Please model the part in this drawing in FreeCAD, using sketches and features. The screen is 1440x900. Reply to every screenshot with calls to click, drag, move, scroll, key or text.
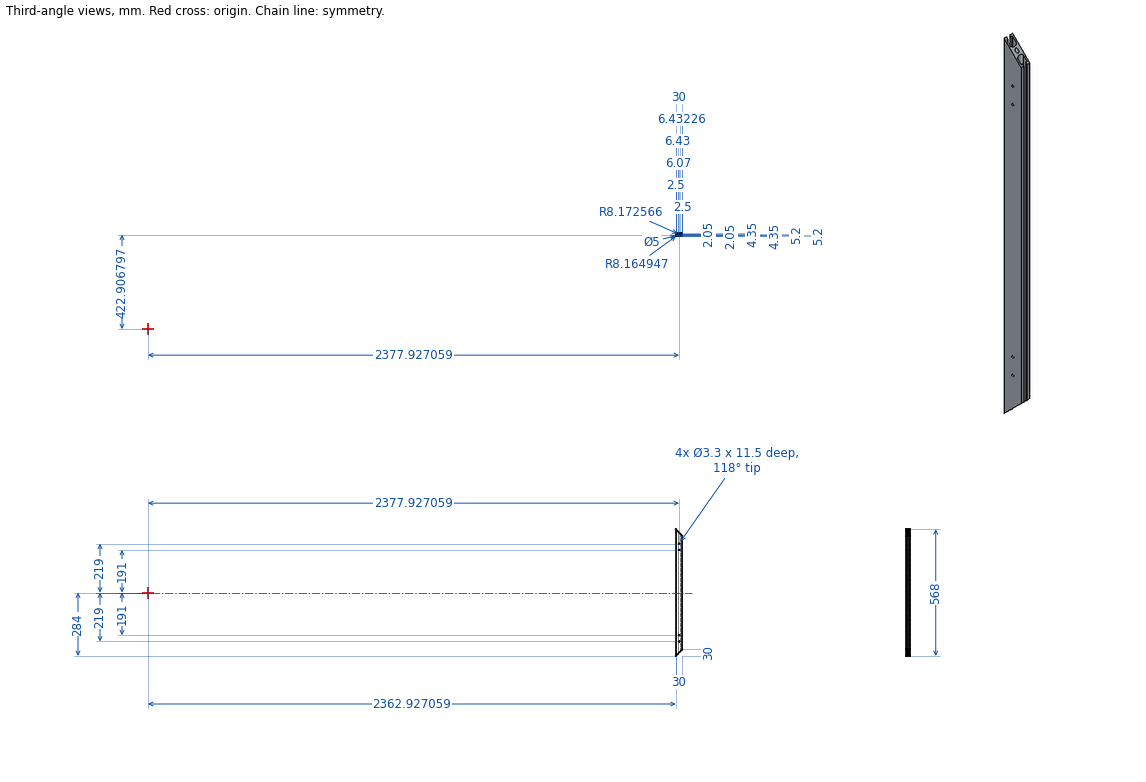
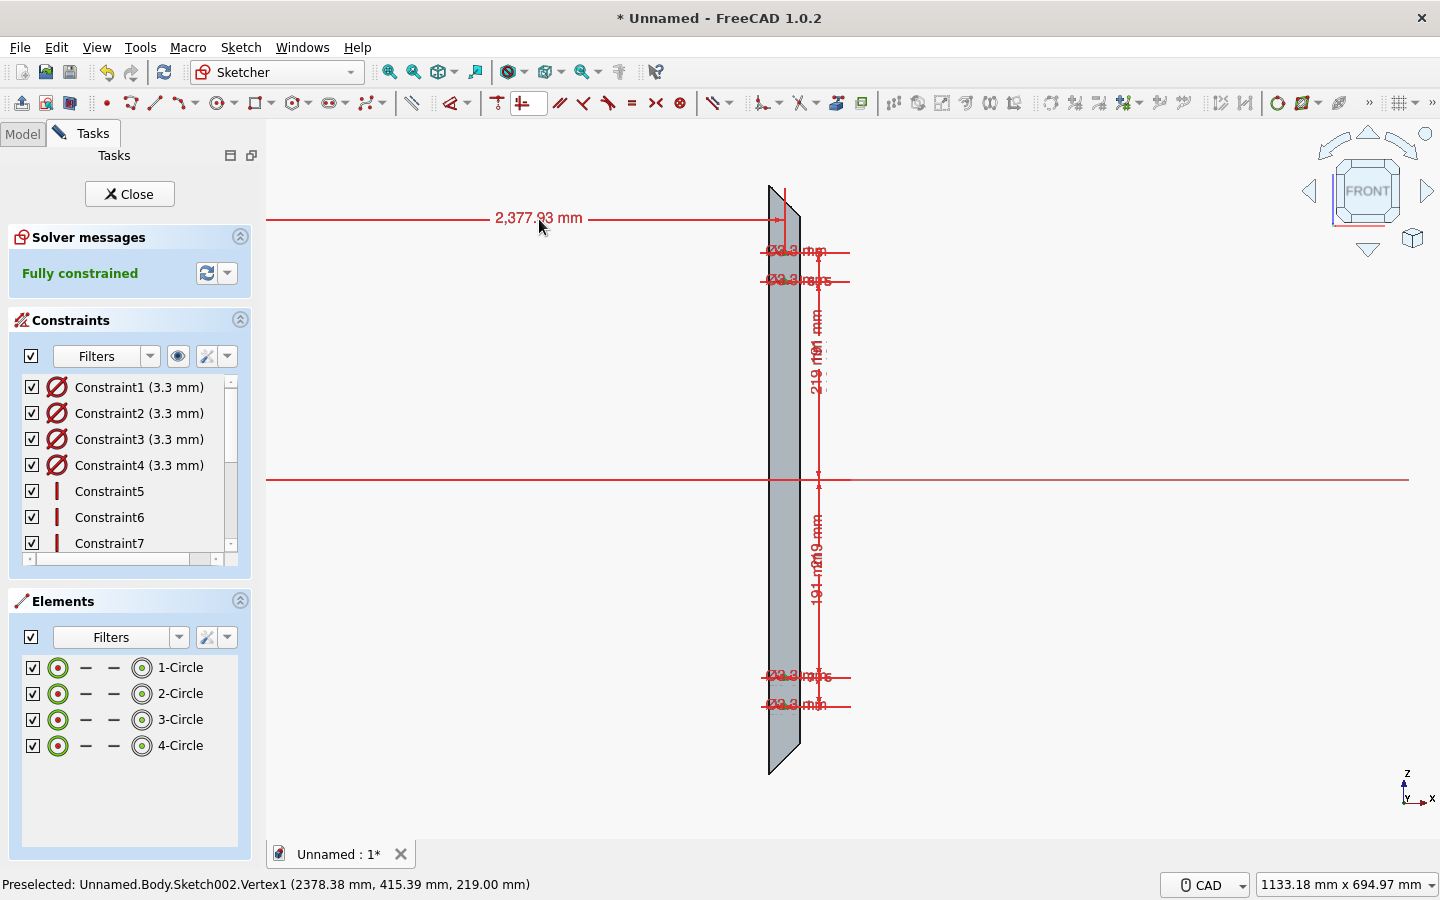
click(130, 194)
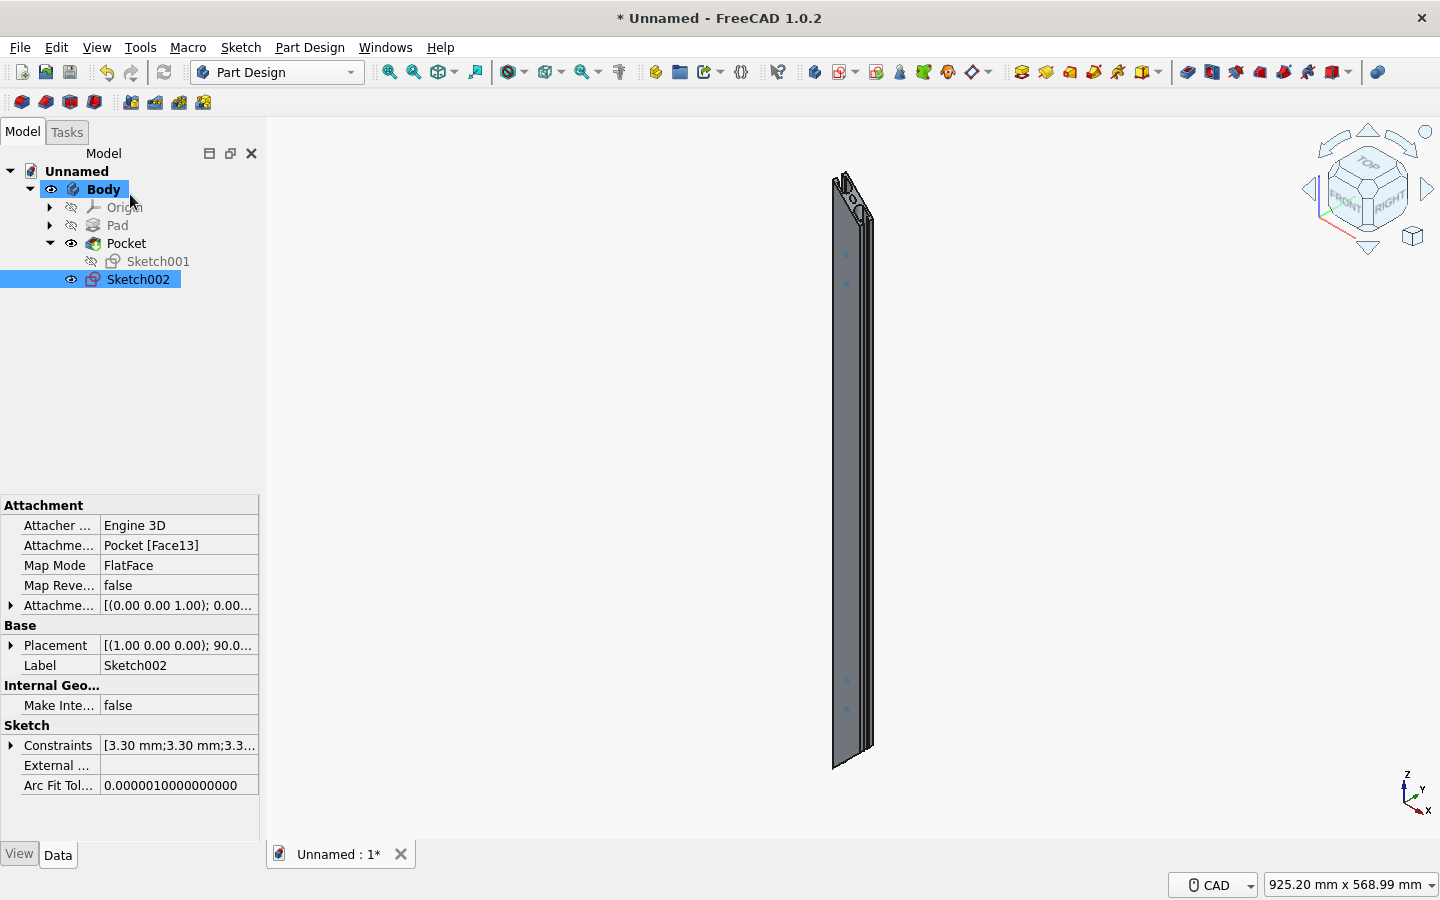
click(1212, 72)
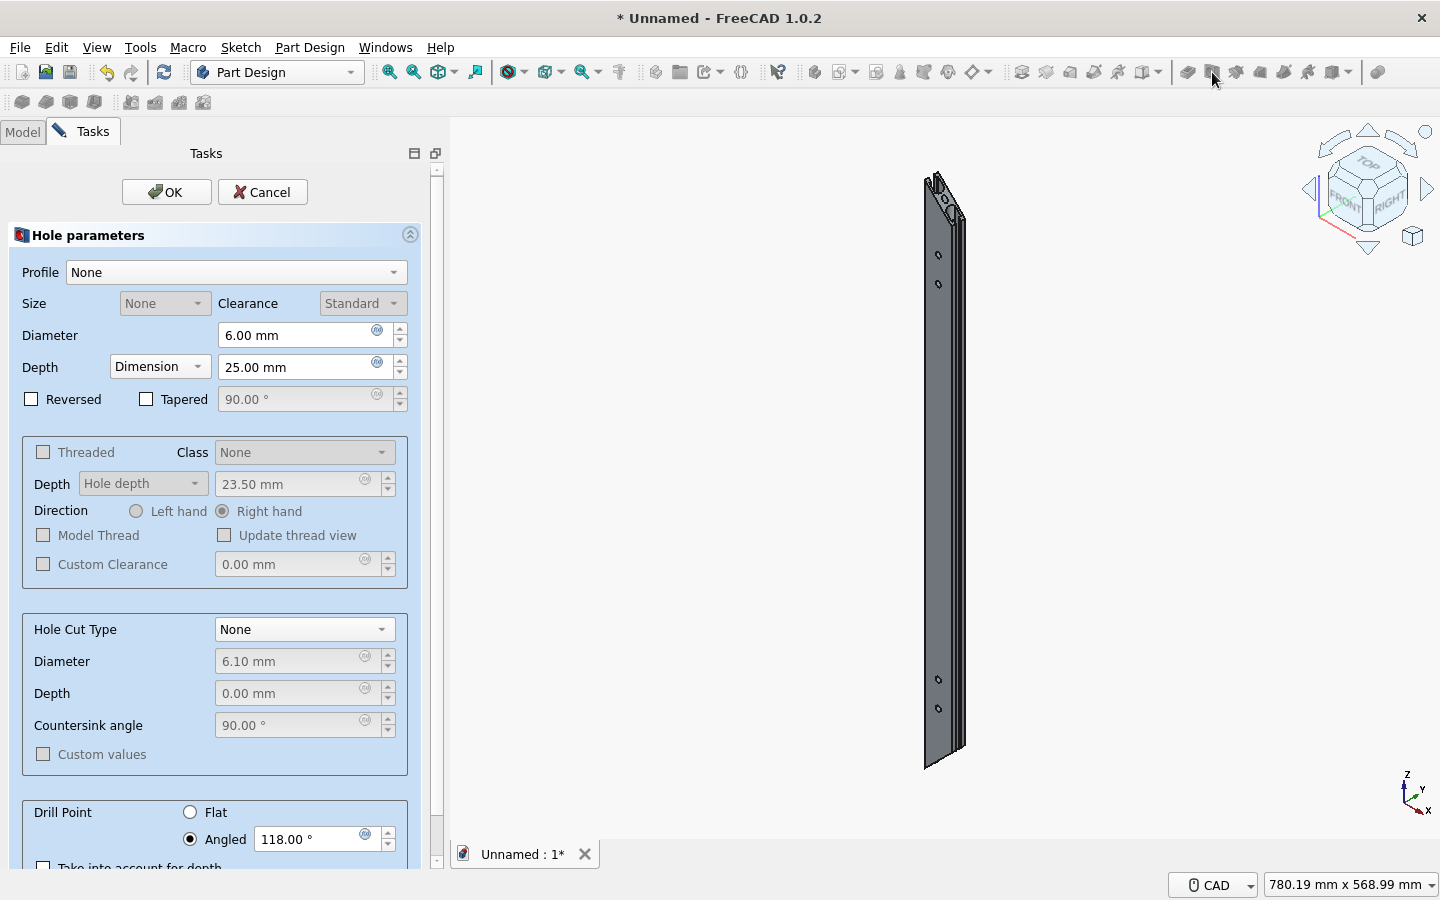
triple_click(305, 335)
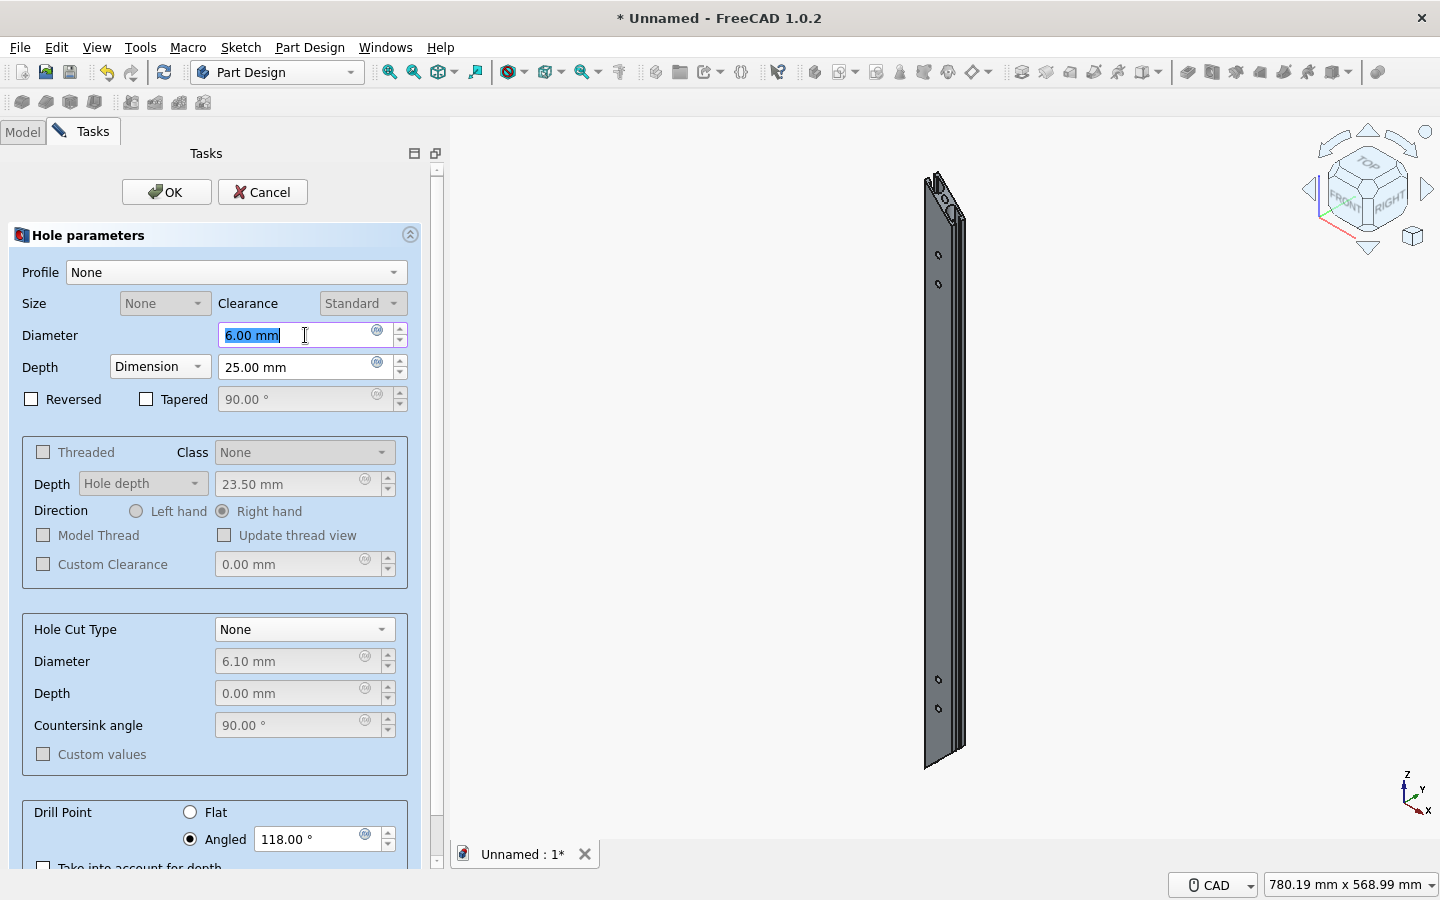
text(3.3)
key(Tab)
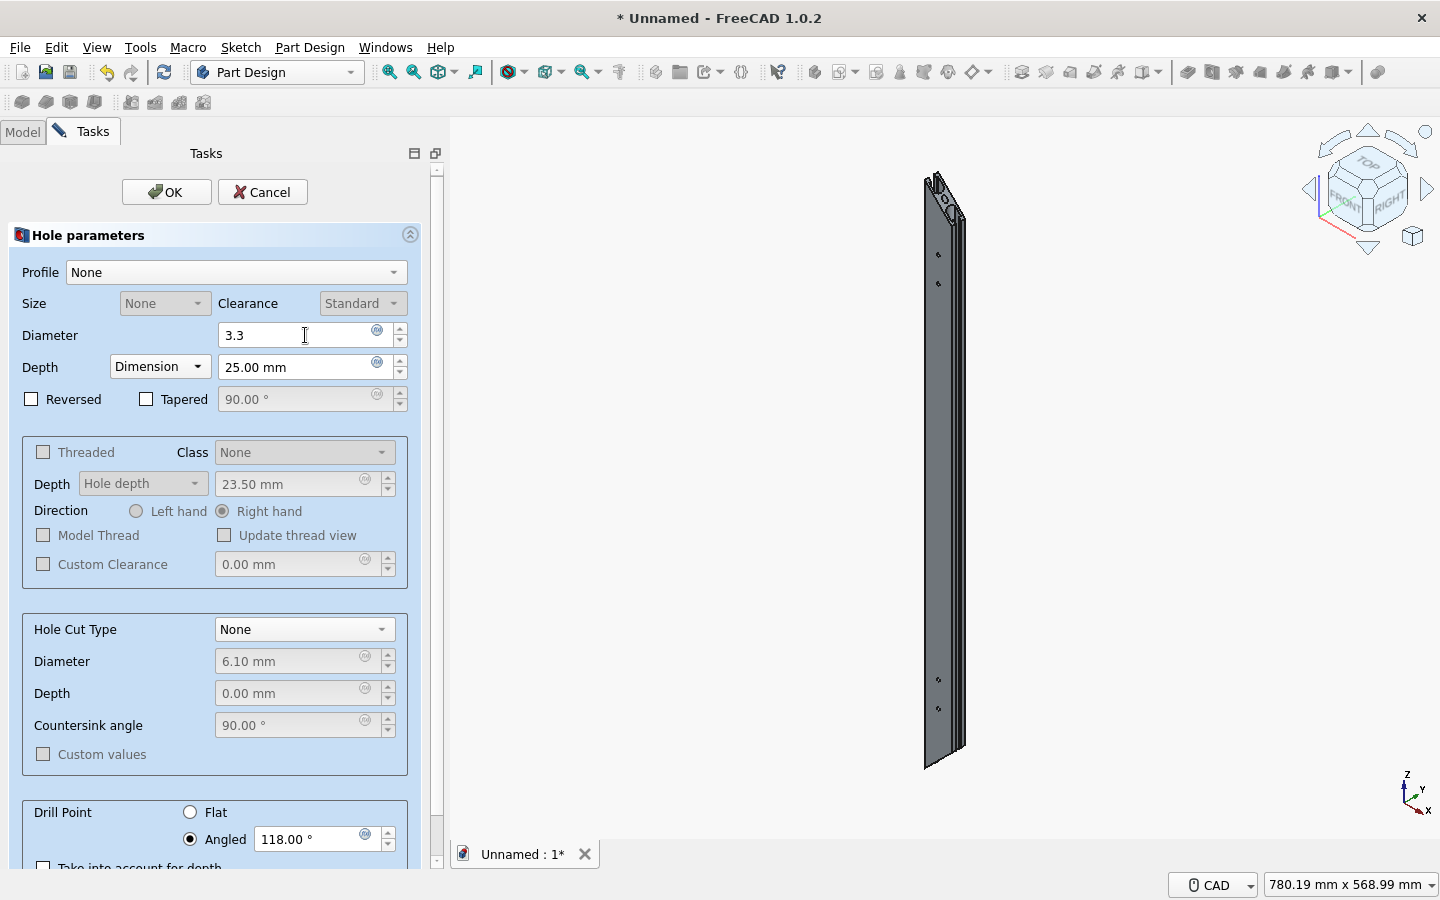
triple_click(305, 367)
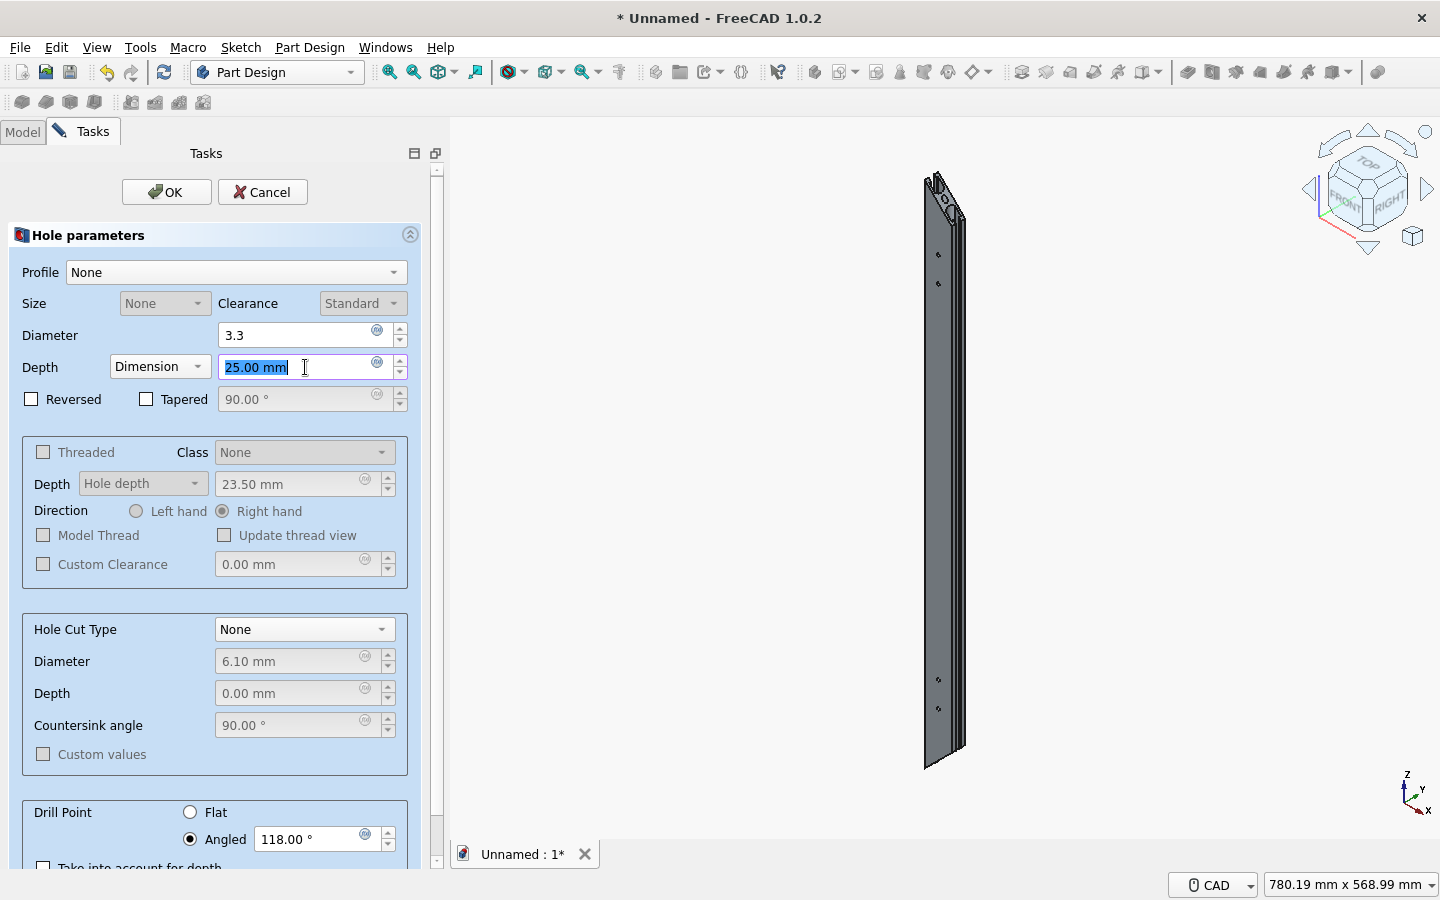
text(11.5)
key(Tab)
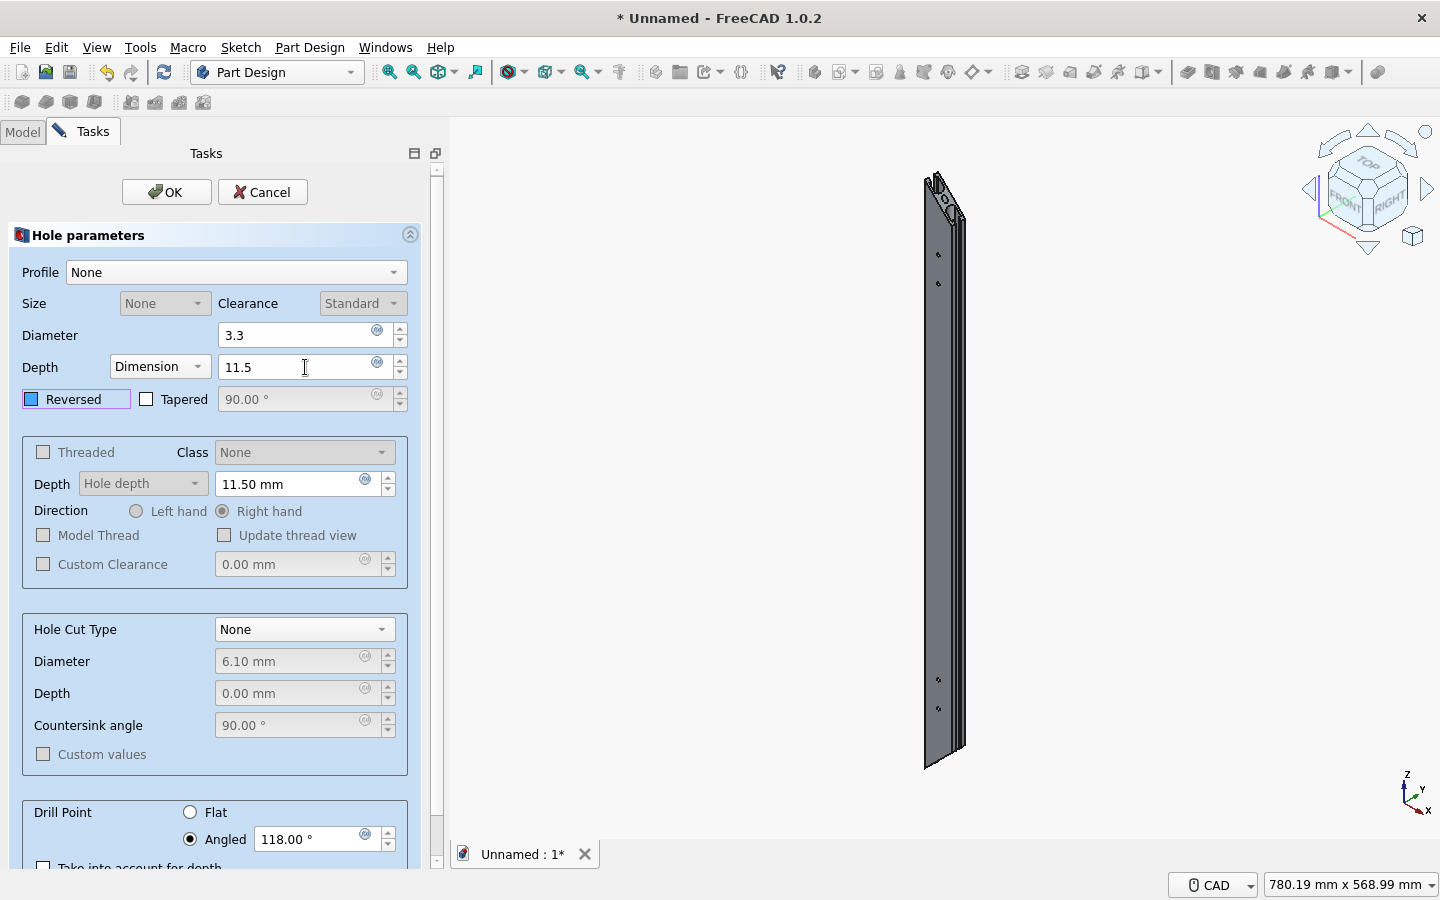
click(167, 192)